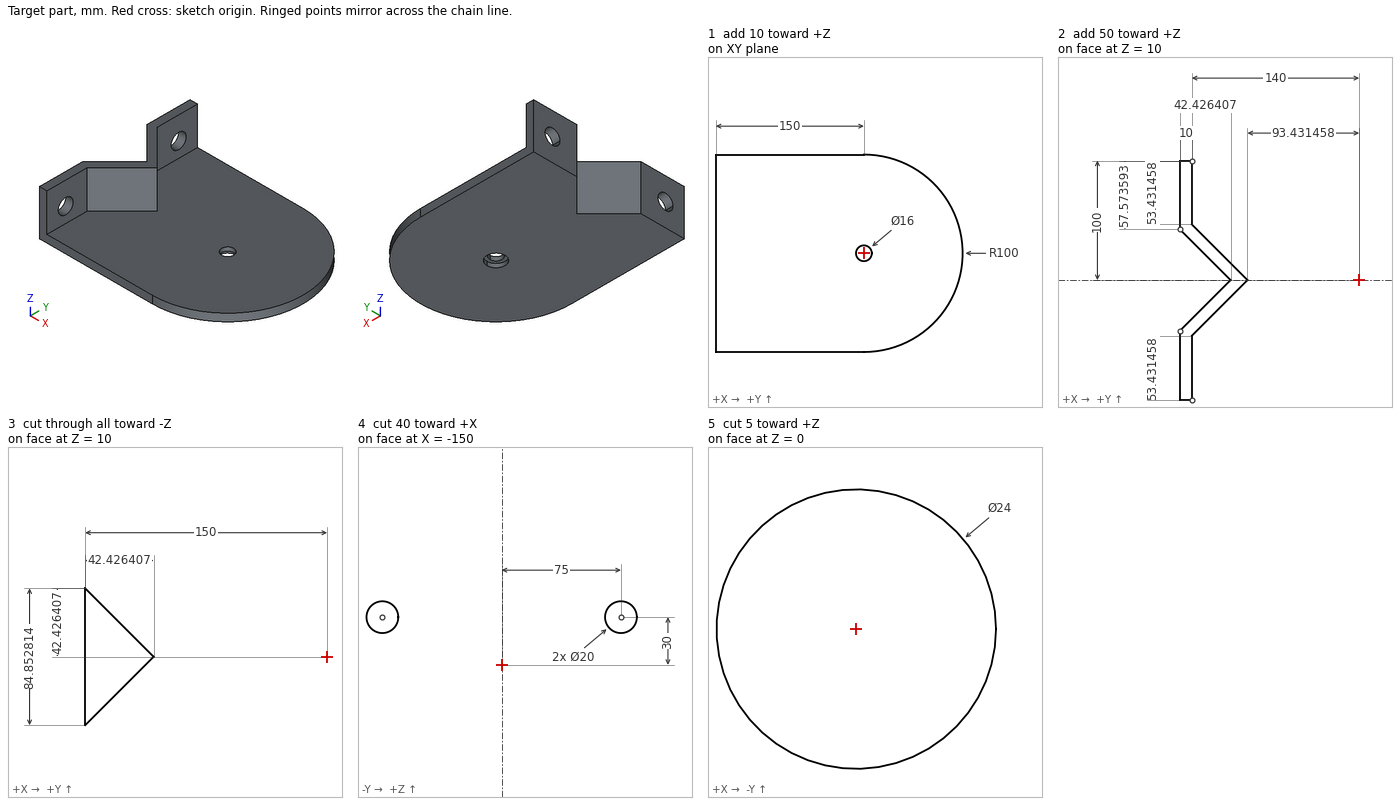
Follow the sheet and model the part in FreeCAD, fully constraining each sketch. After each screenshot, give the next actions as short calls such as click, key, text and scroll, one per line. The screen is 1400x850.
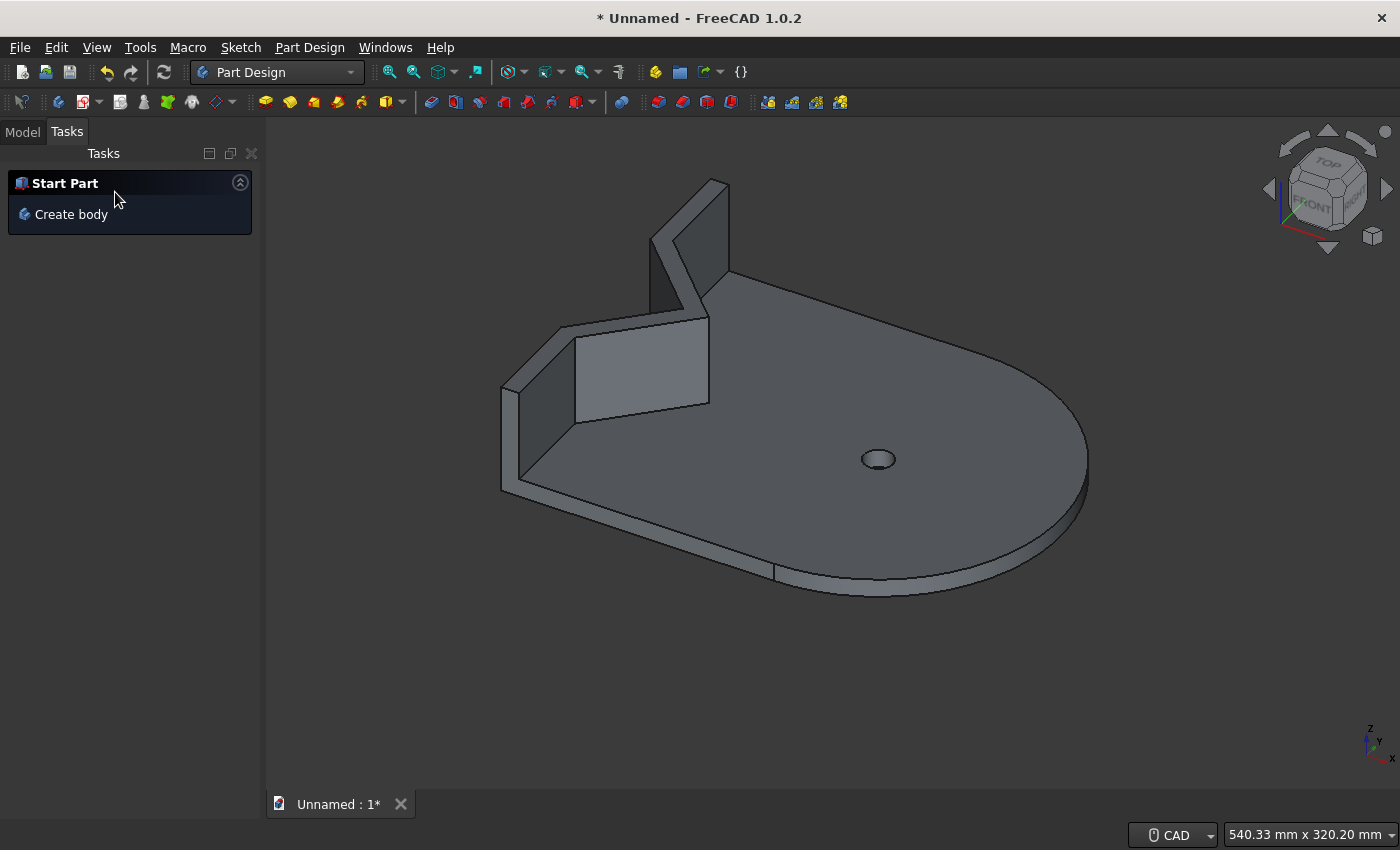
click(810, 396)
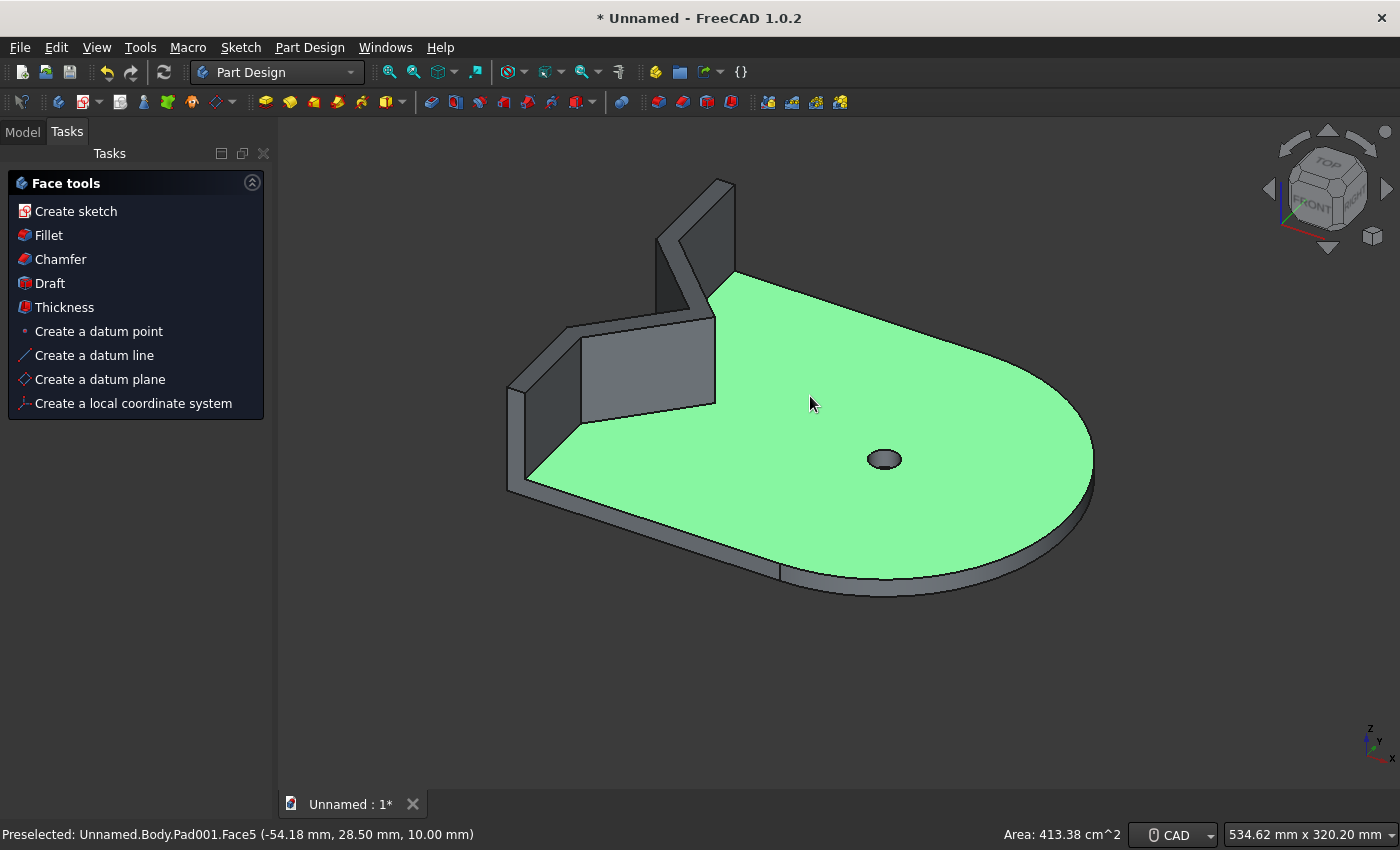
click(84, 102)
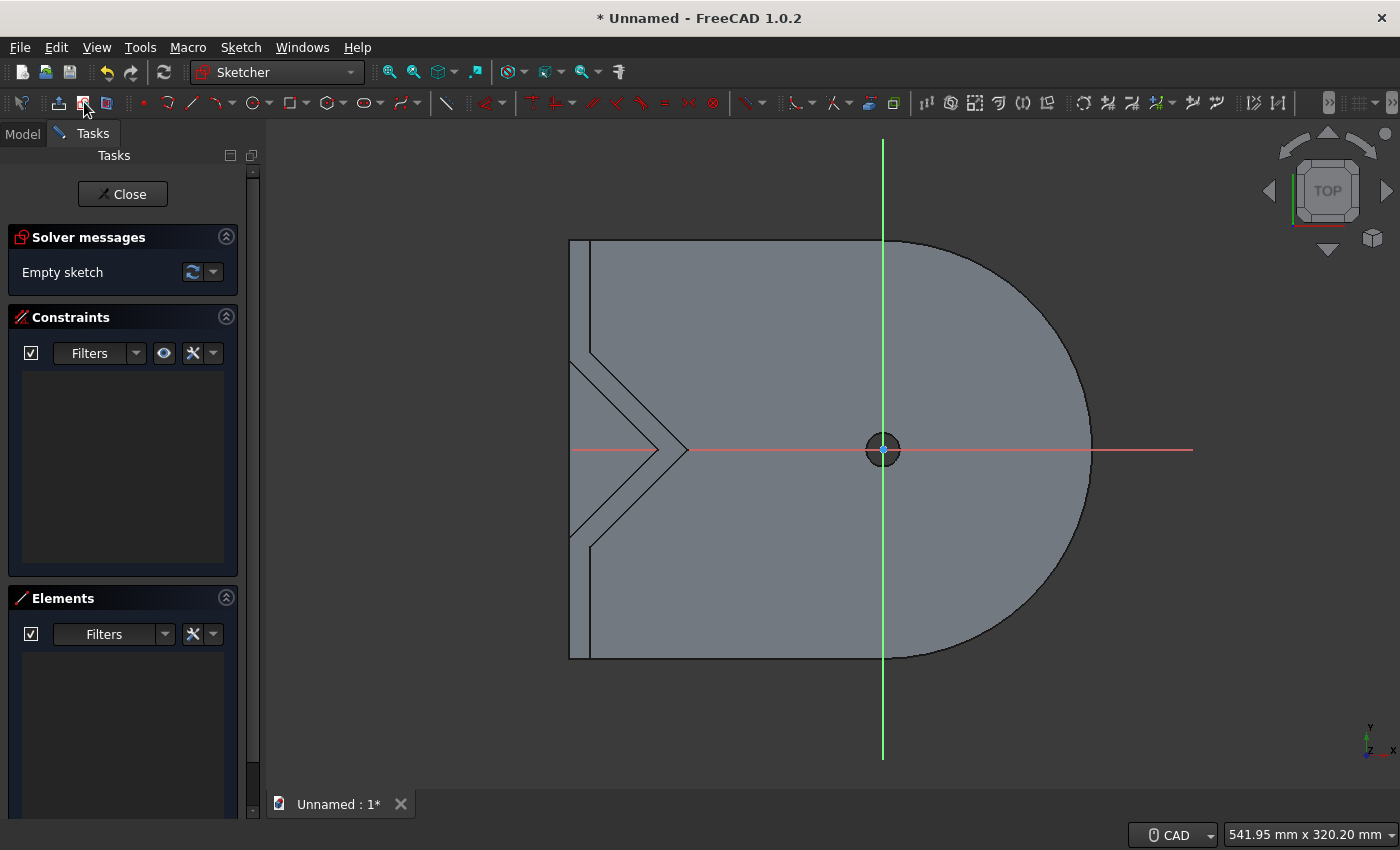
key(q)
key(s)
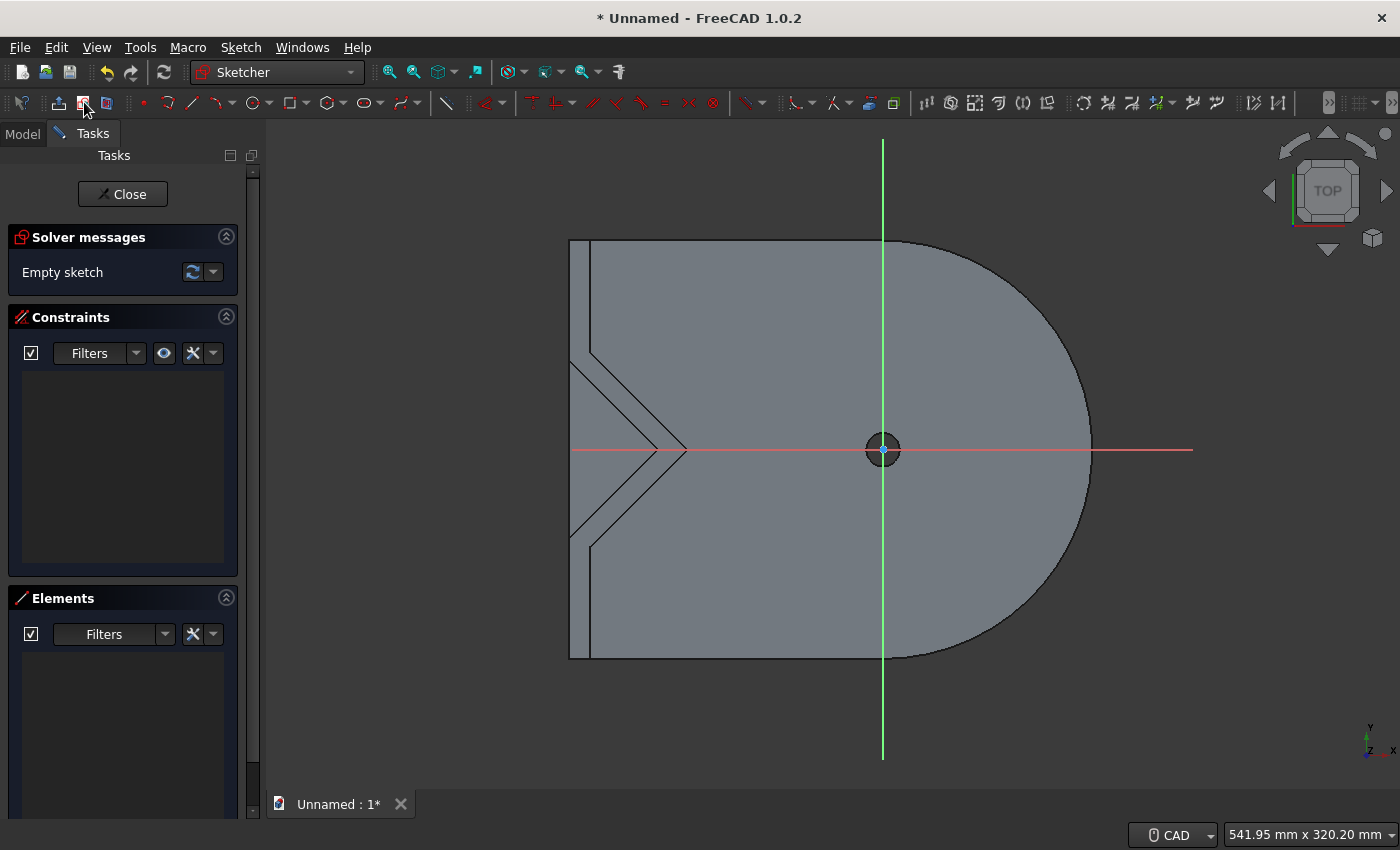
scroll(695, 446, up, 4)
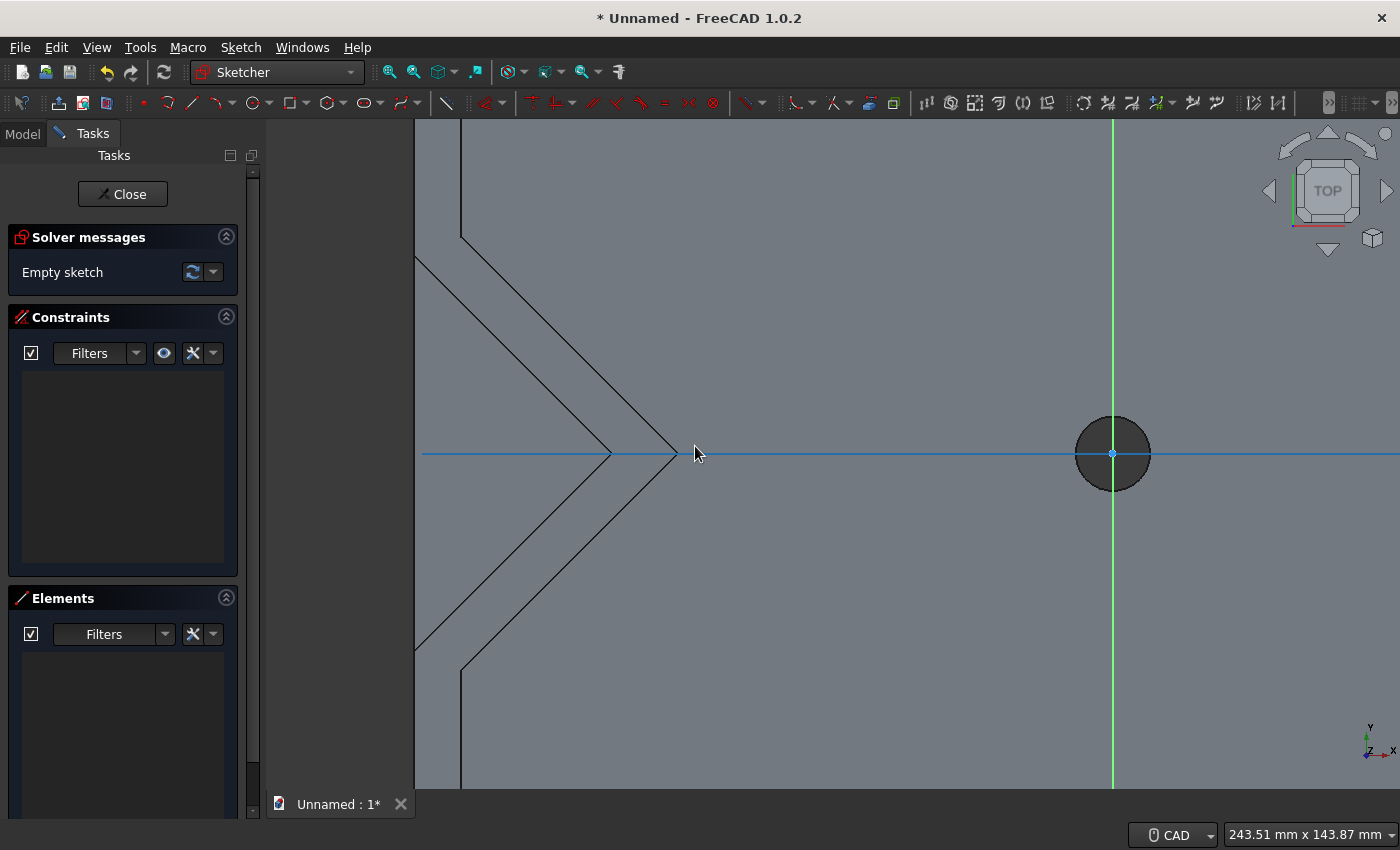
click(168, 104)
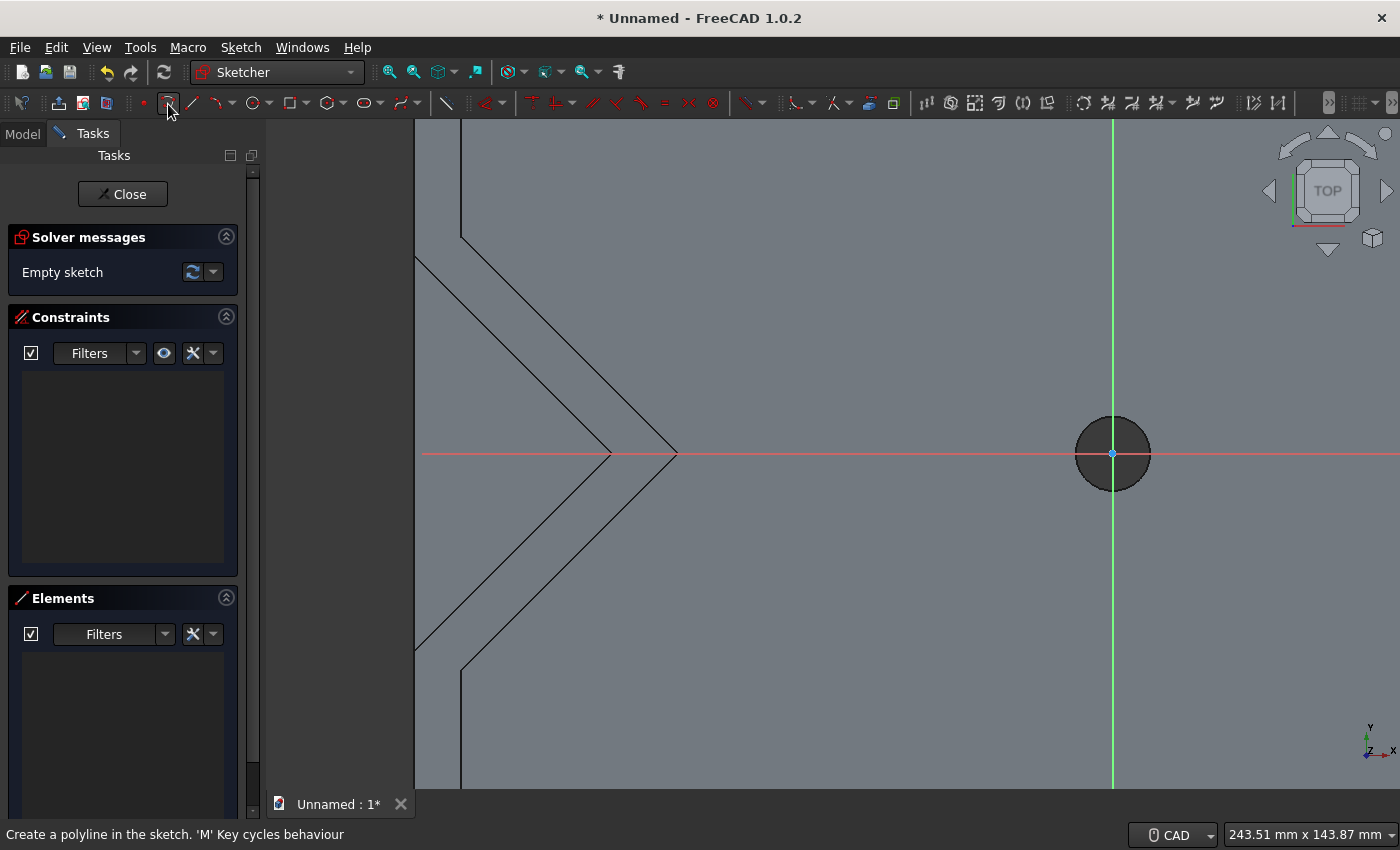
click(612, 454)
click(414, 256)
click(414, 651)
click(612, 454)
key(Escape)
key(Escape)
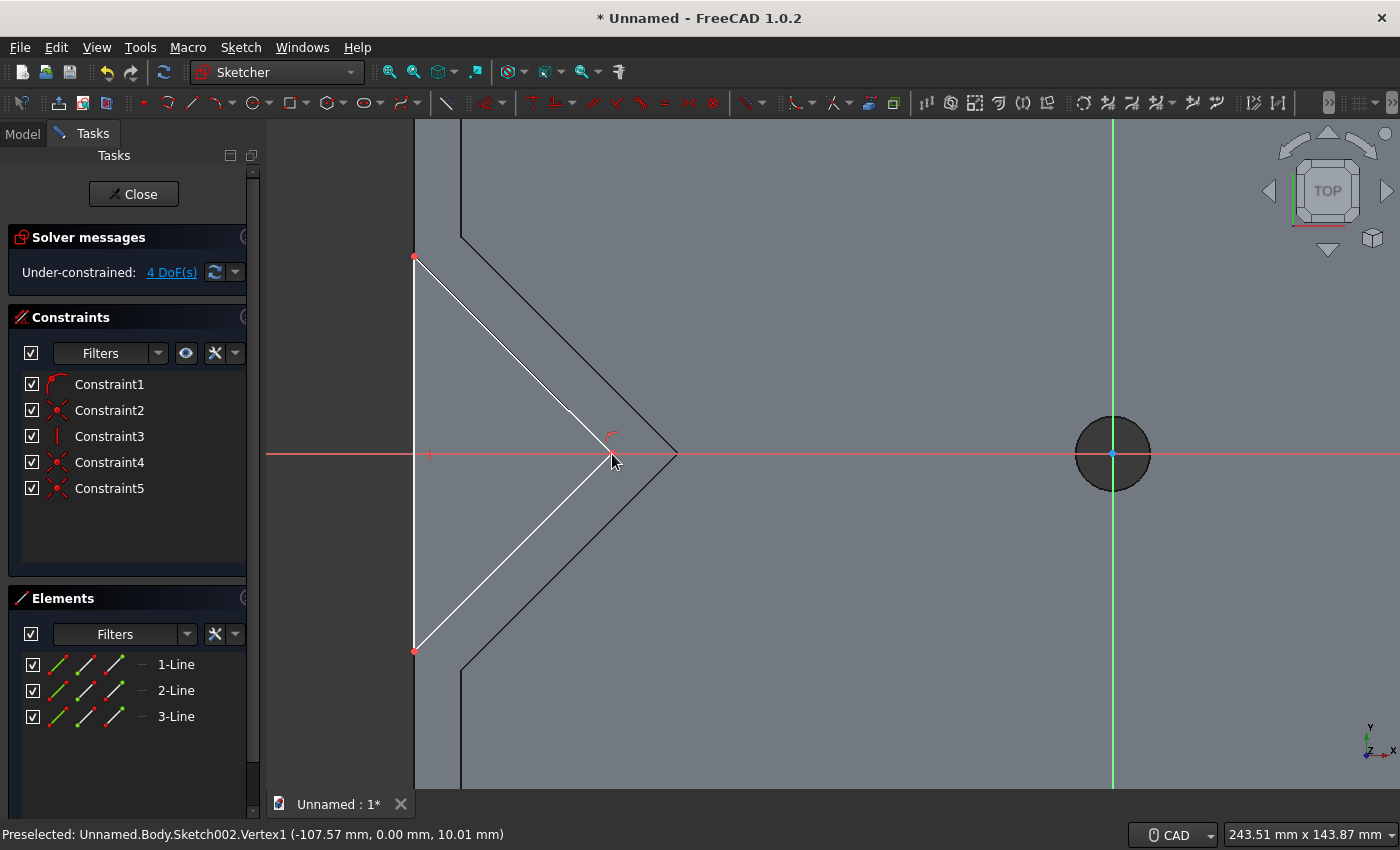
click(486, 104)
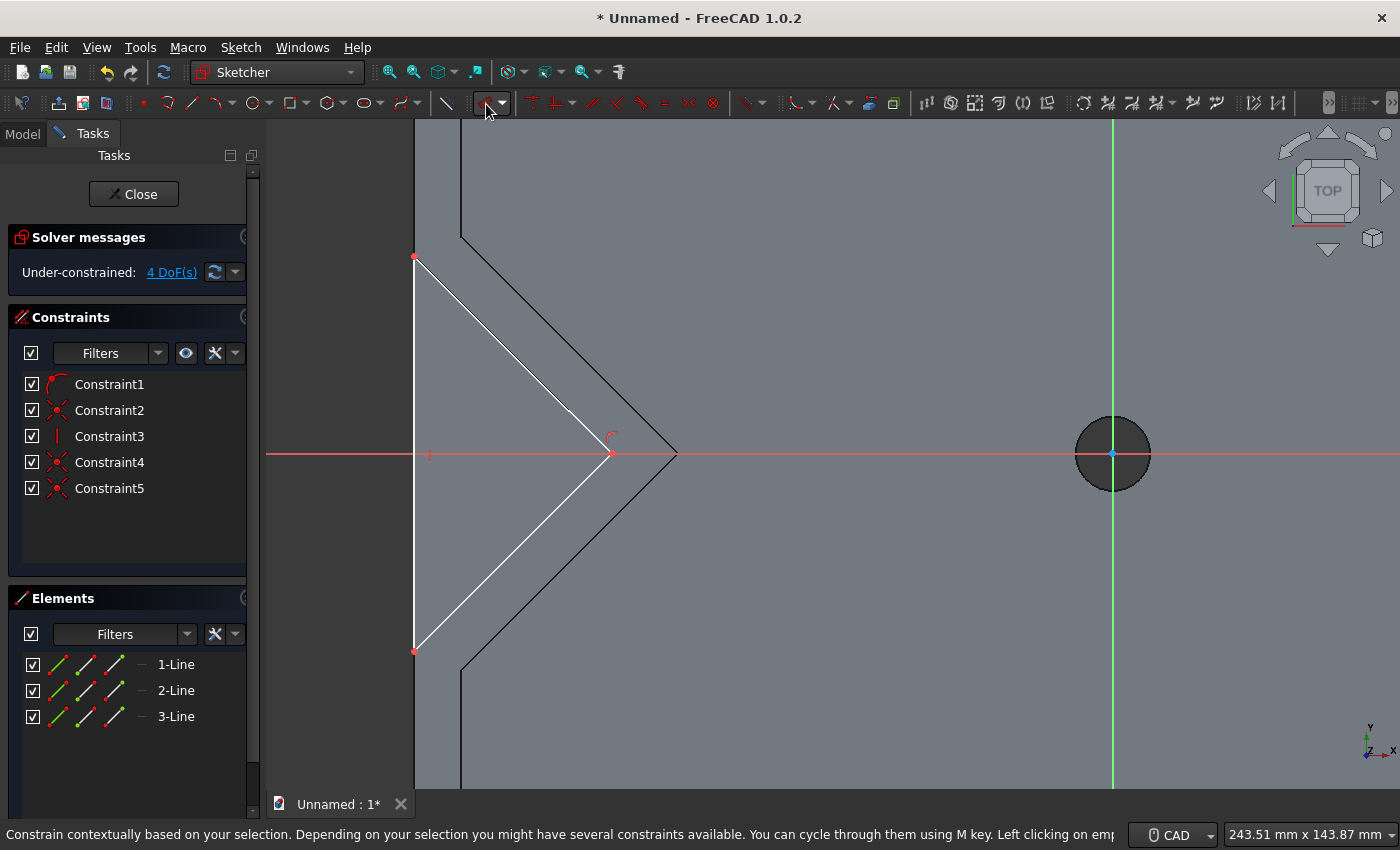
click(414, 257)
click(763, 223)